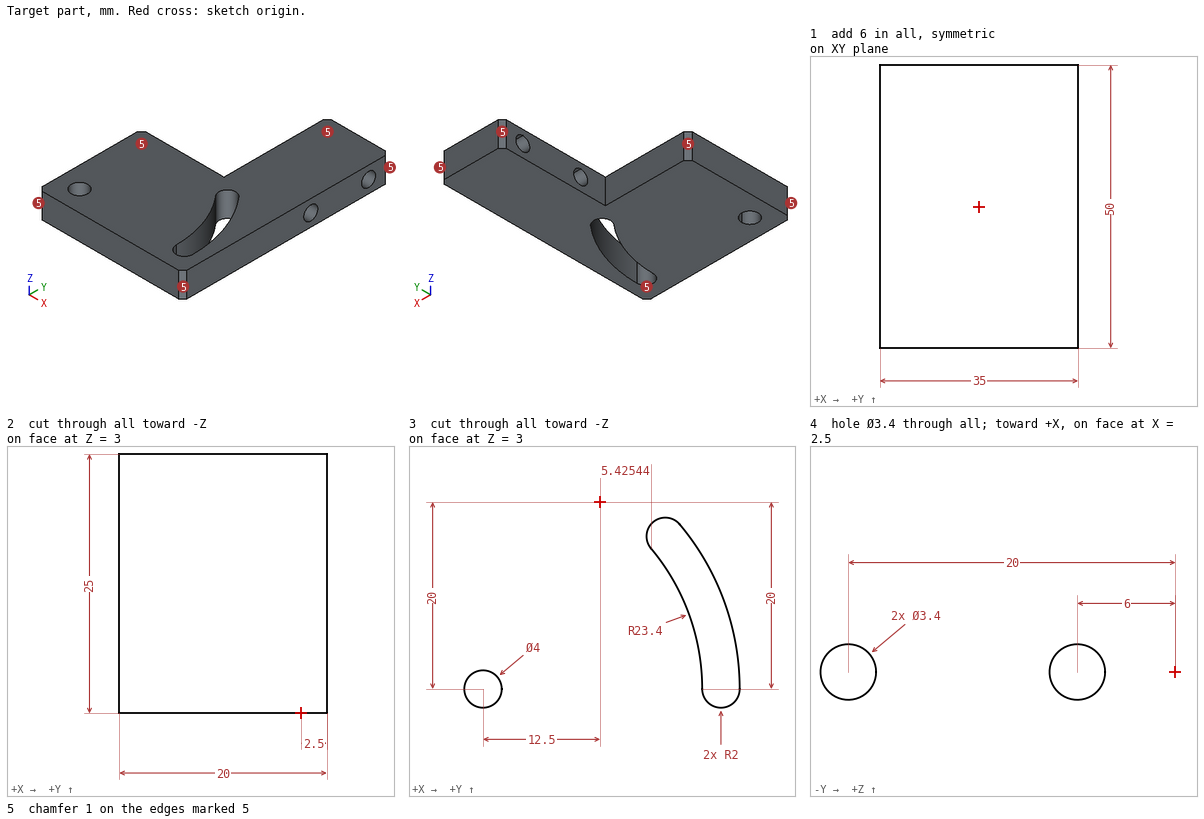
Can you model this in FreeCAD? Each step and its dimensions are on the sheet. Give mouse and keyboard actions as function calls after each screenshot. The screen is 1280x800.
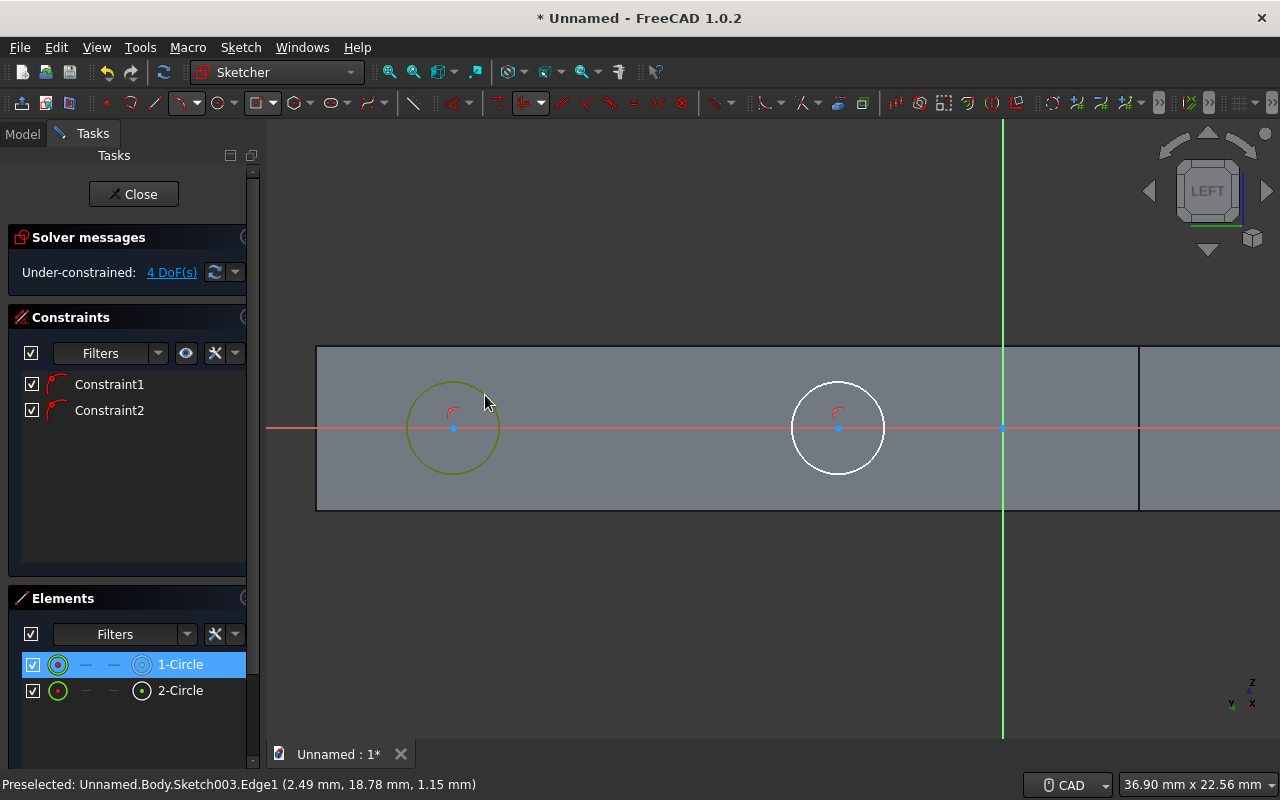
click(870, 395)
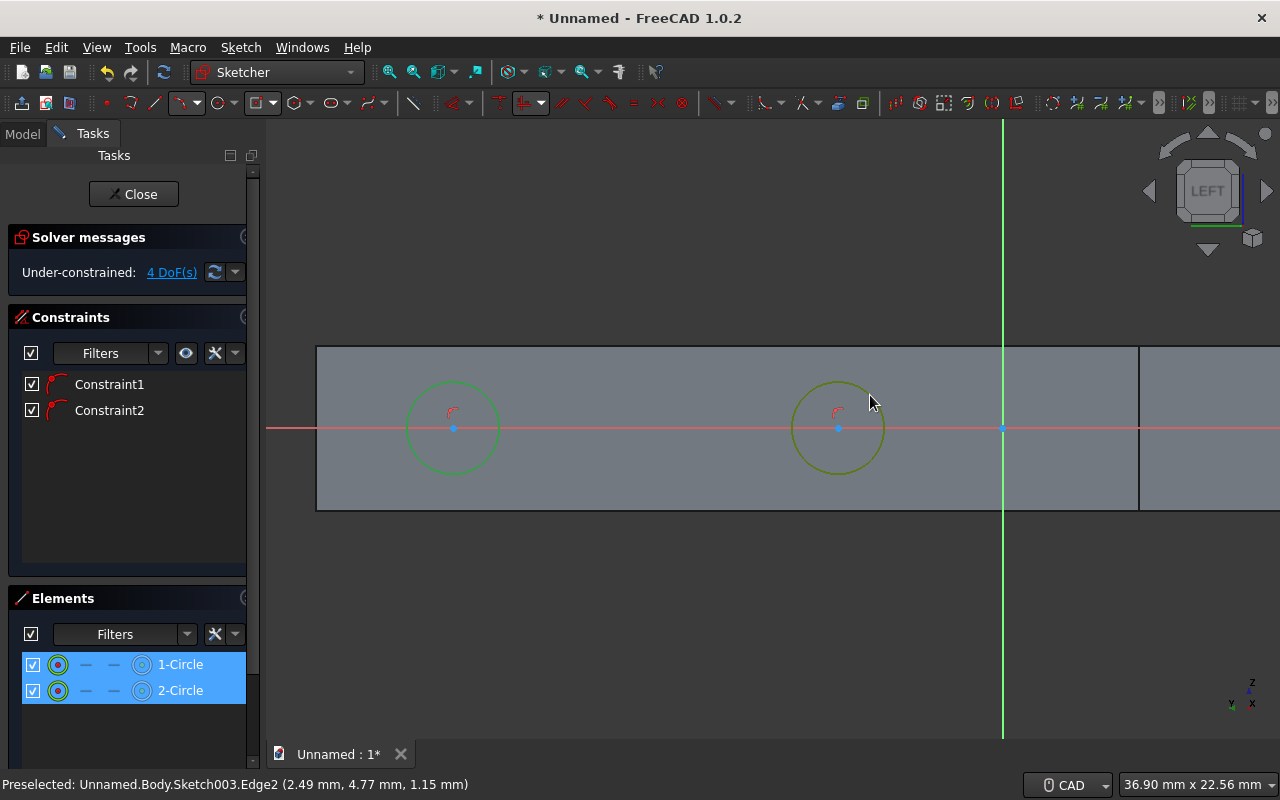
click(634, 104)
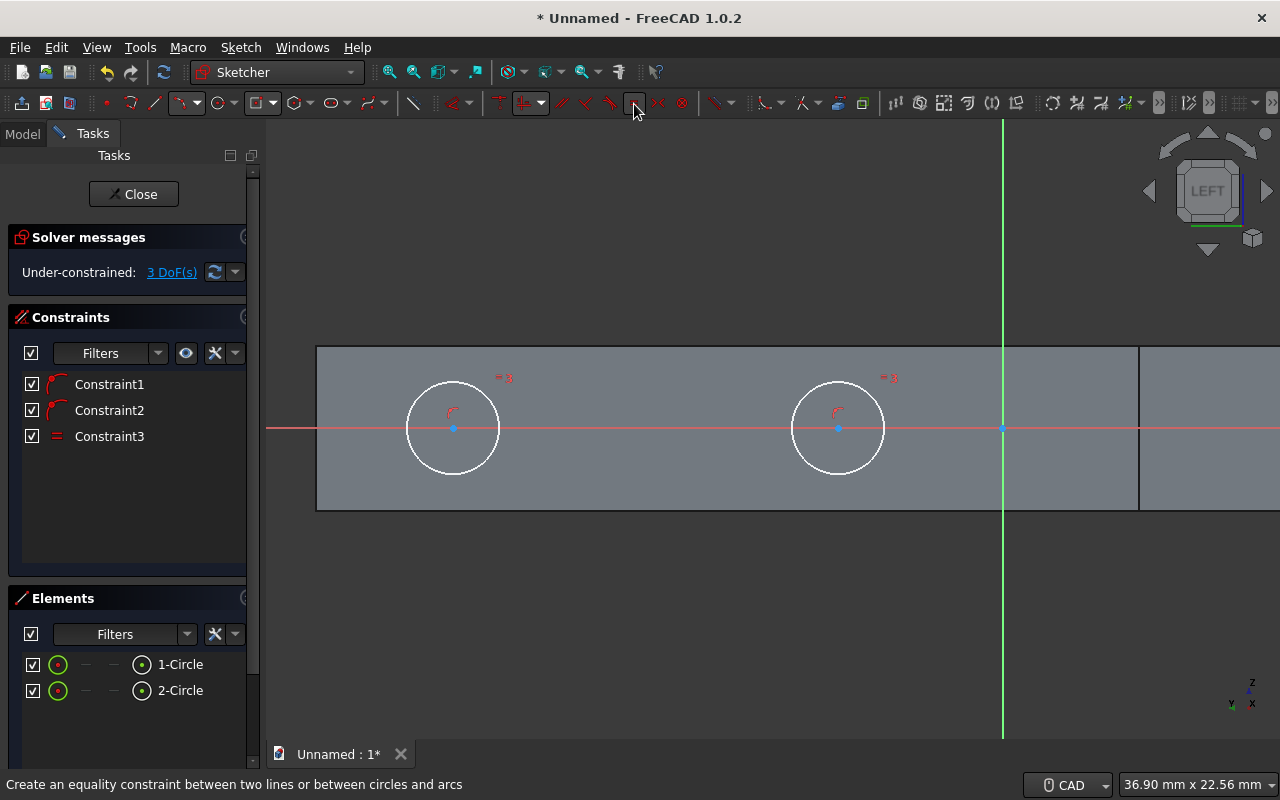
click(452, 104)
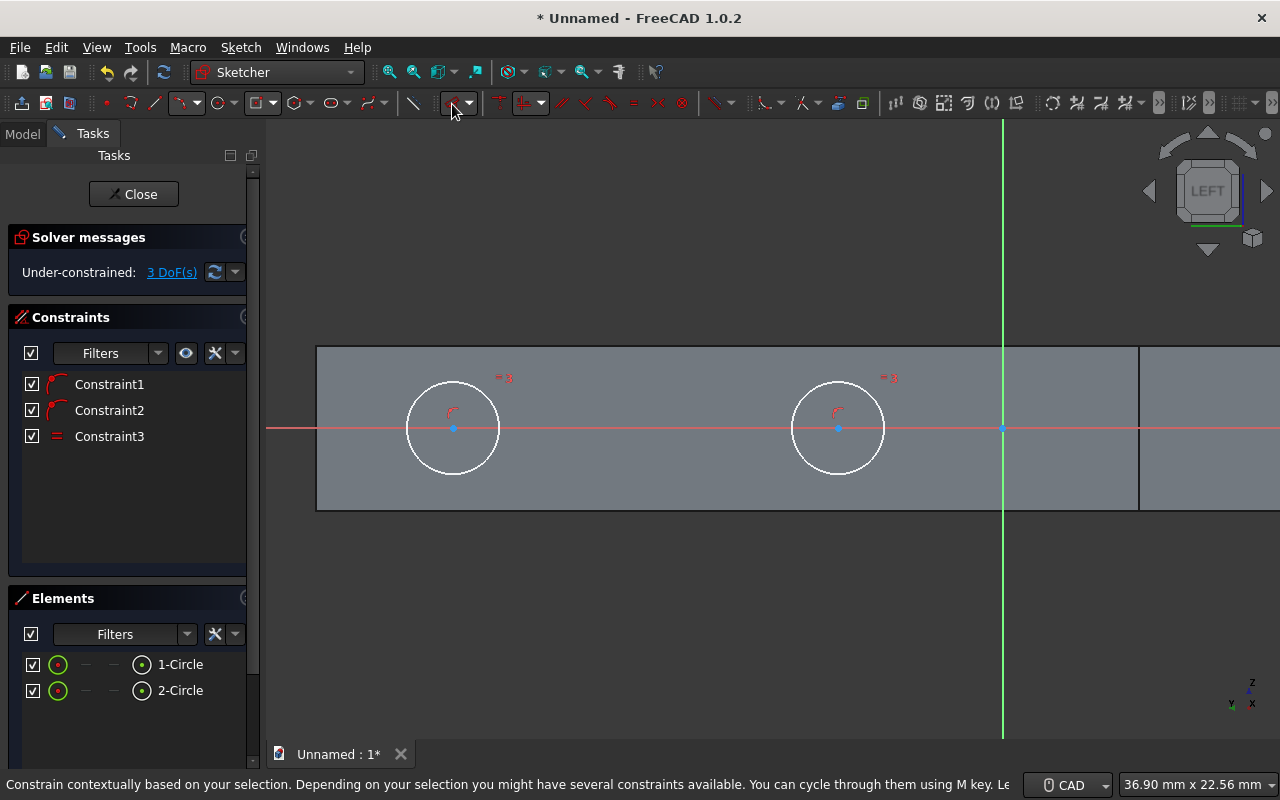
click(485, 395)
click(507, 372)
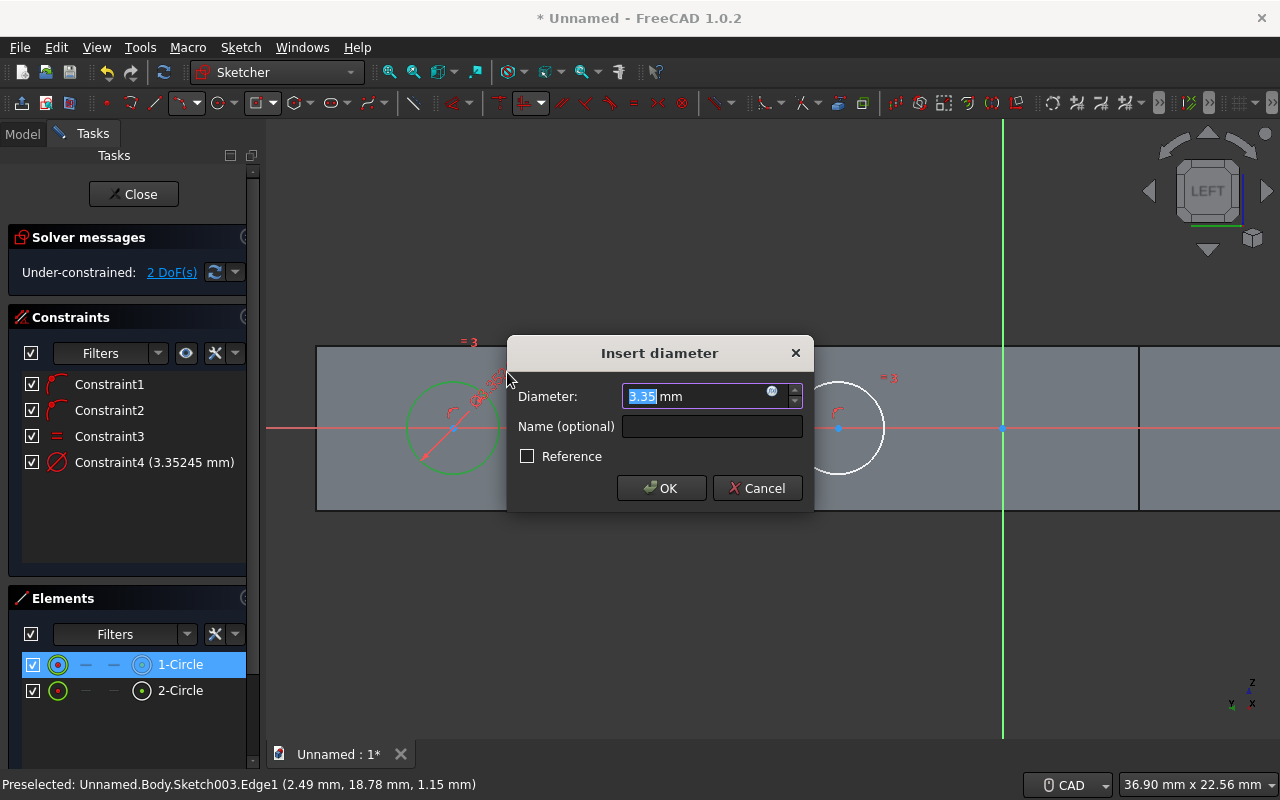
text(3.4)
key(Return)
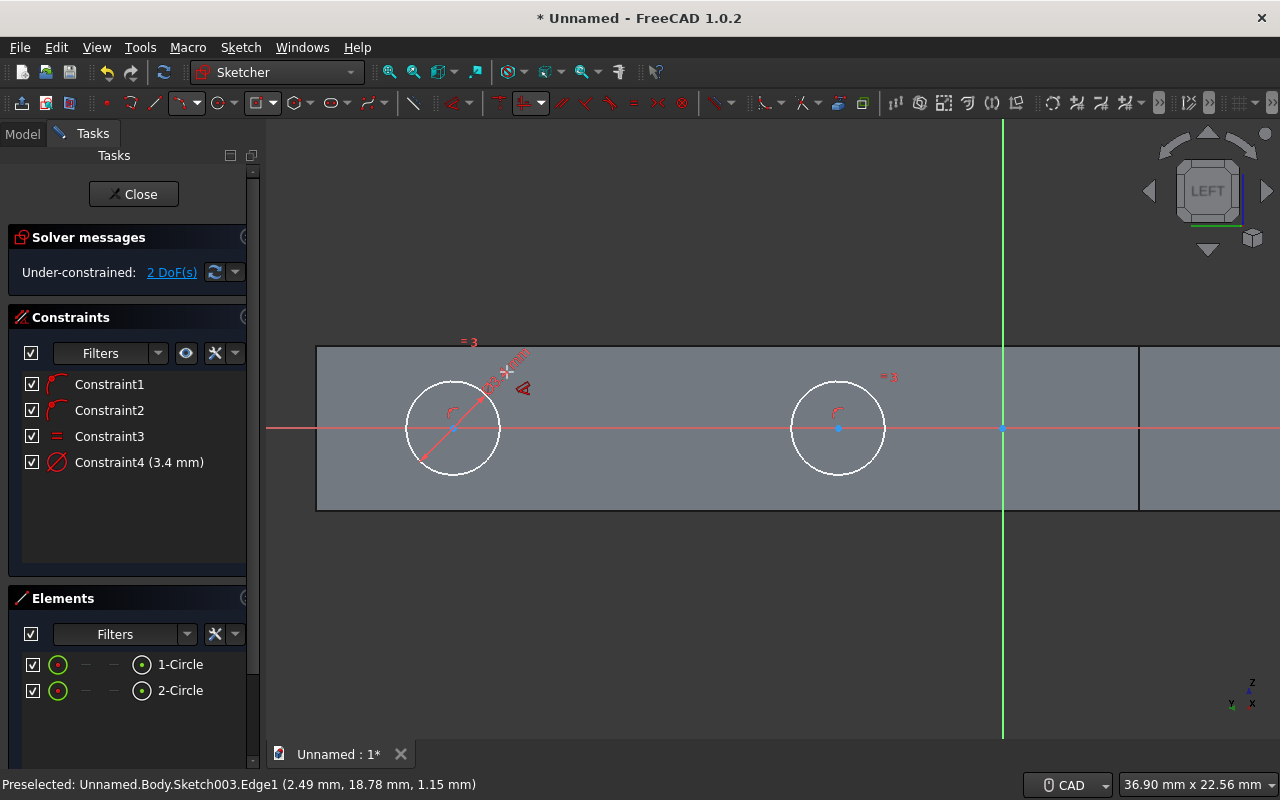
click(838, 428)
click(920, 462)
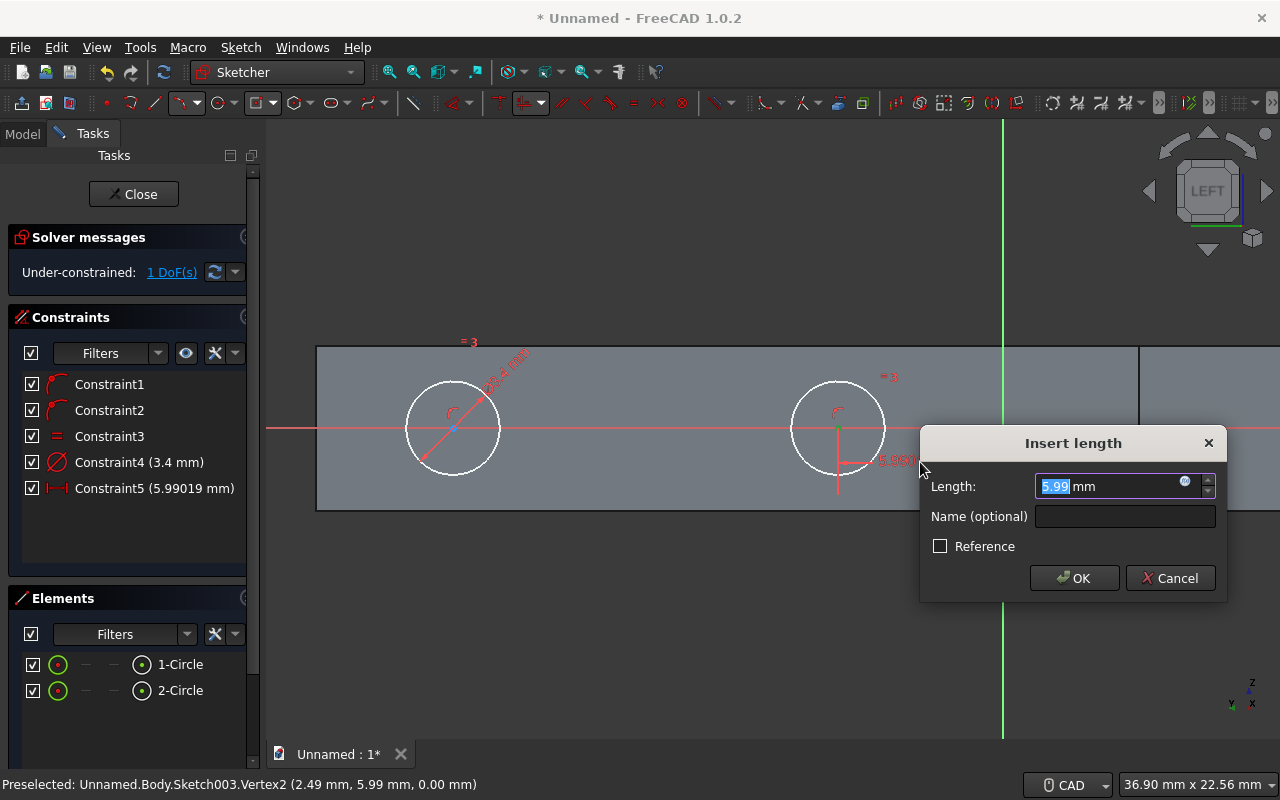
text(6)
key(Return)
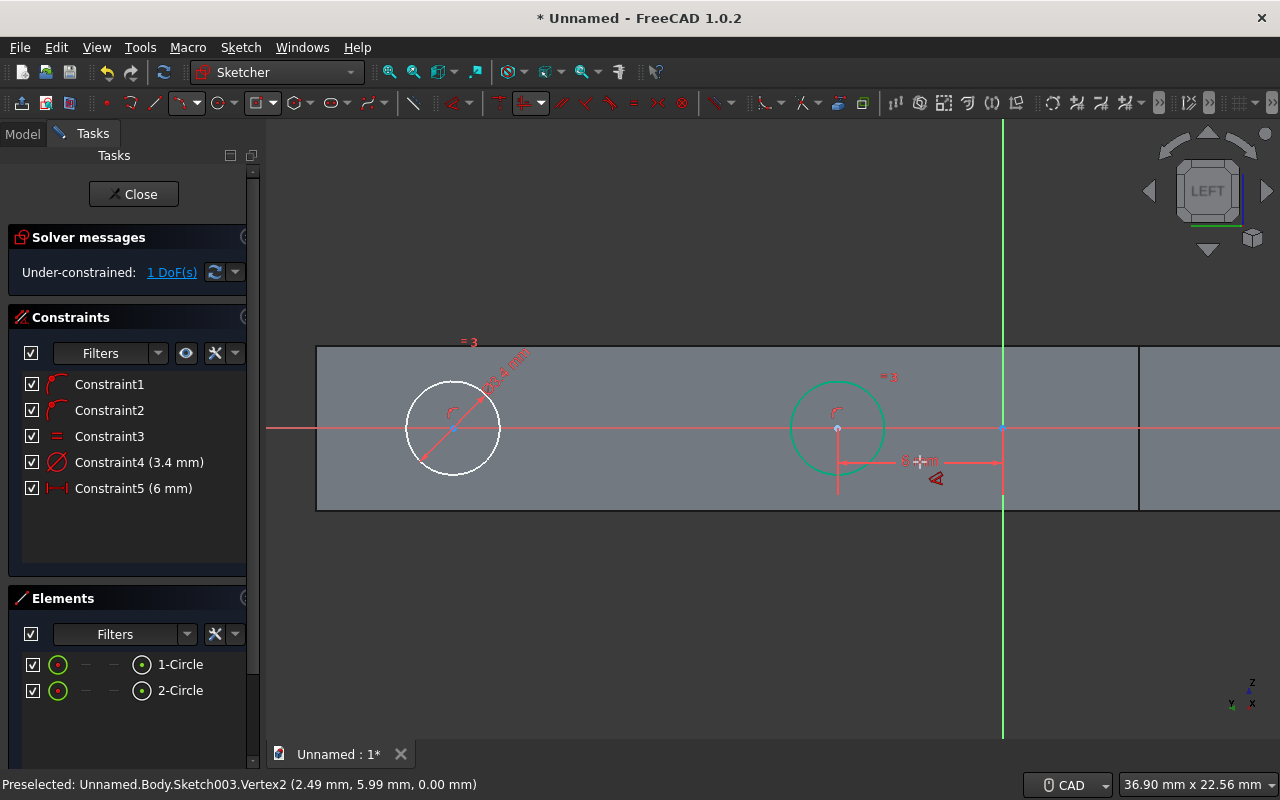
click(453, 428)
click(728, 462)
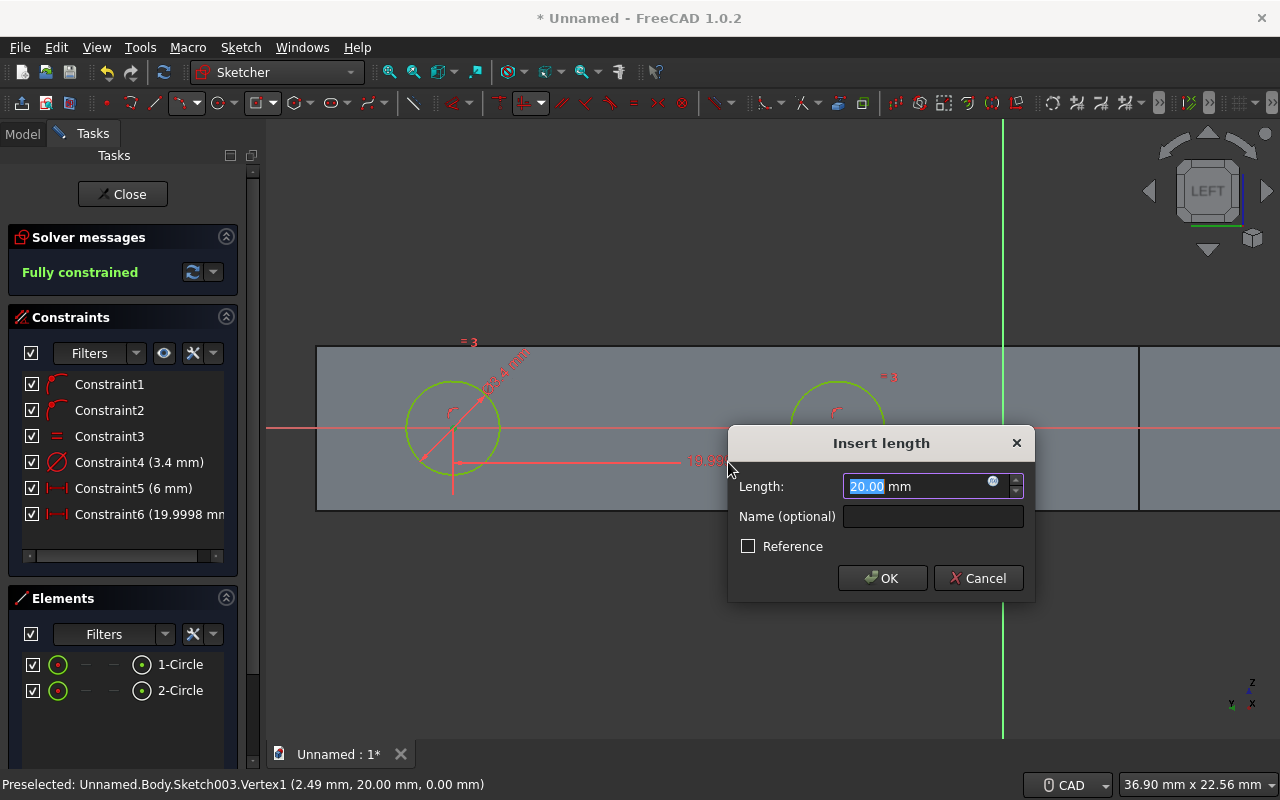
text(20)
key(Return)
key(Escape)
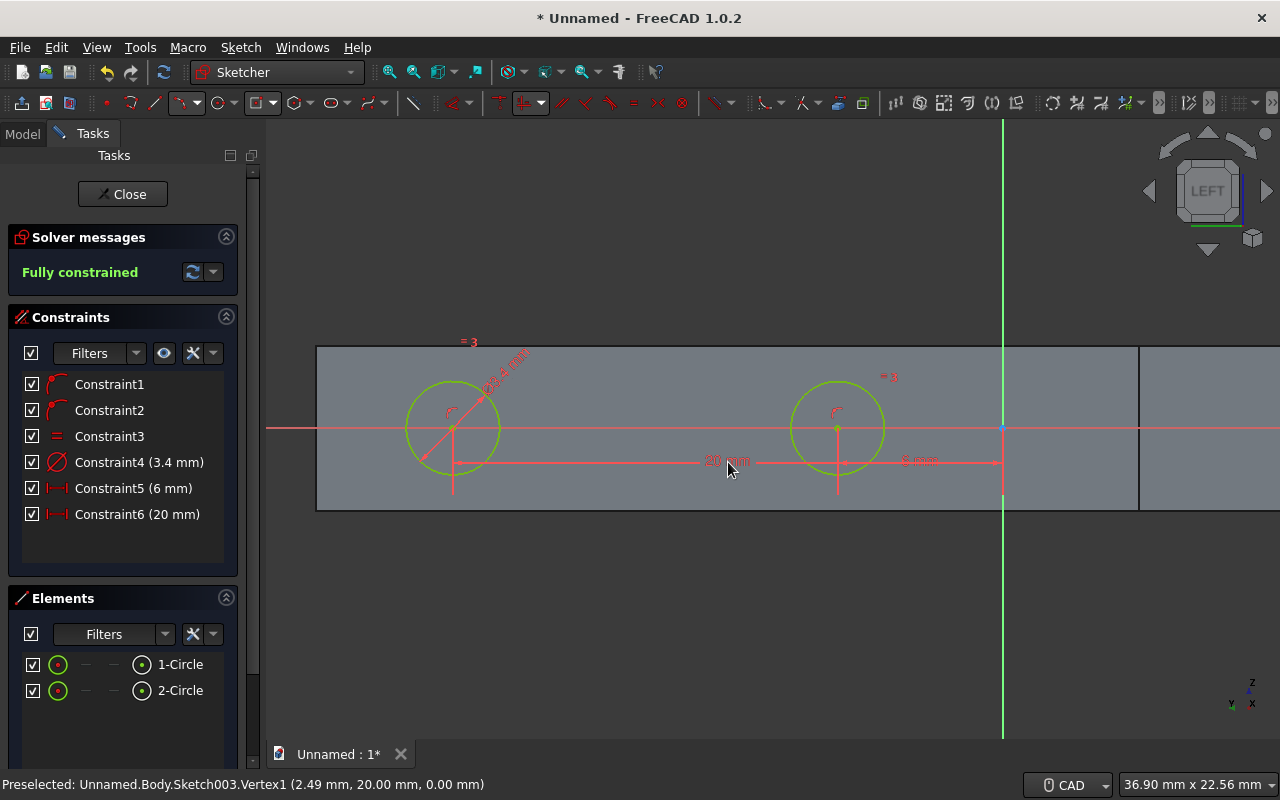
click(123, 194)